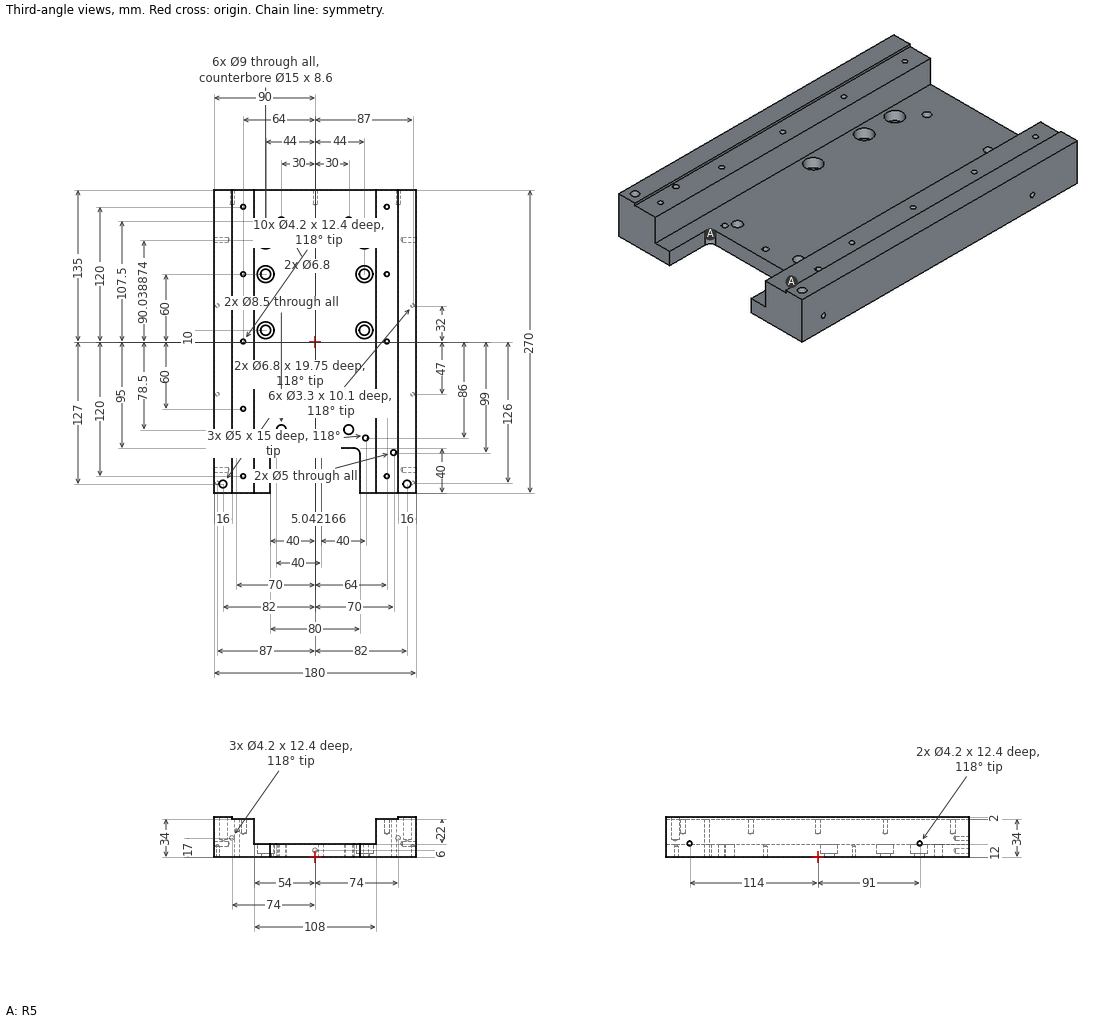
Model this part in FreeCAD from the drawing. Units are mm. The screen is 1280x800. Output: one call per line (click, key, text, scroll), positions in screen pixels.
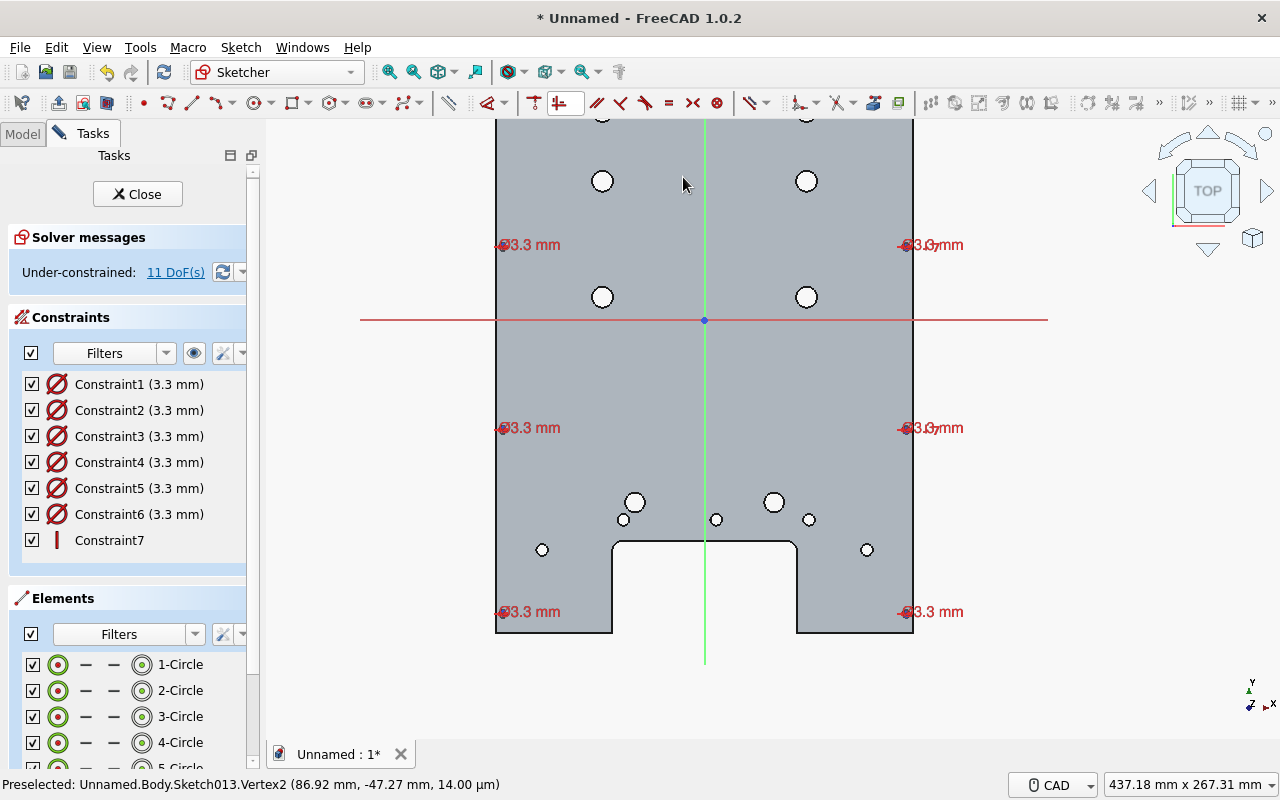
click(906, 430)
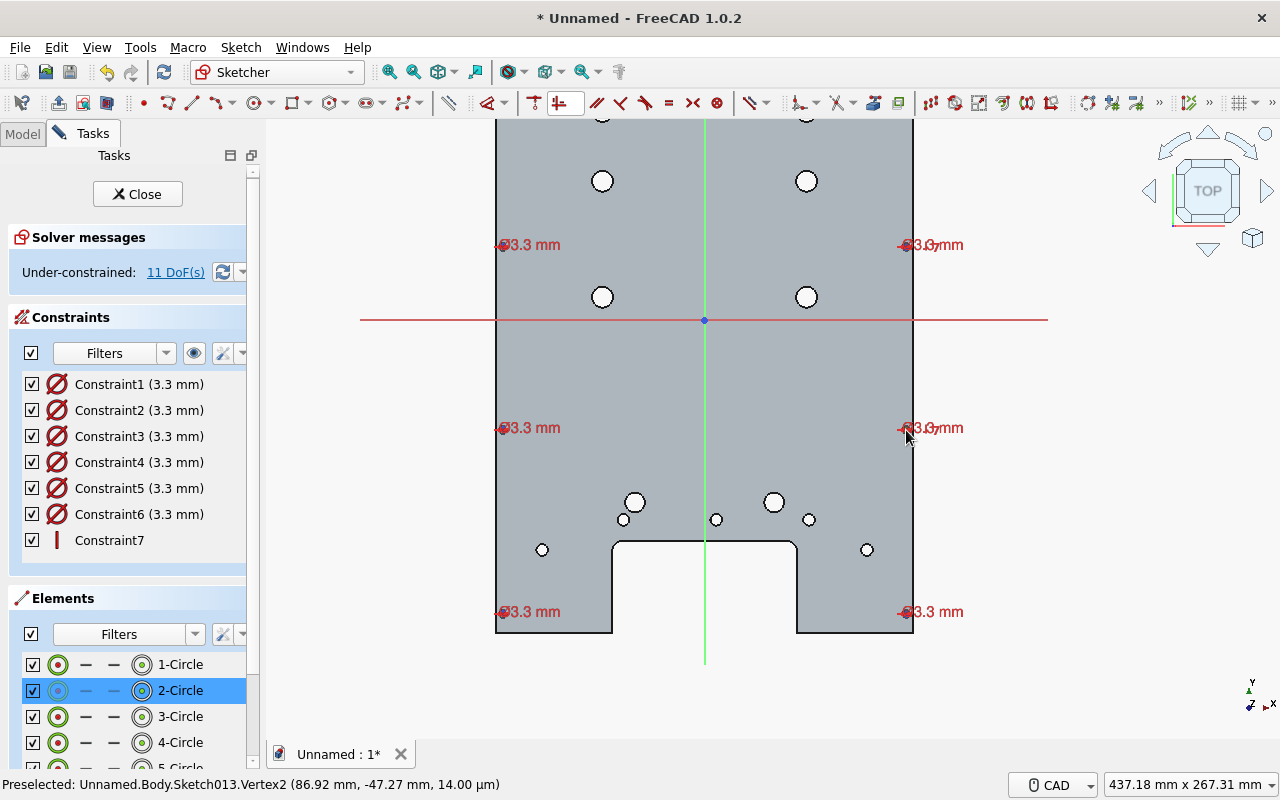
click(906, 614)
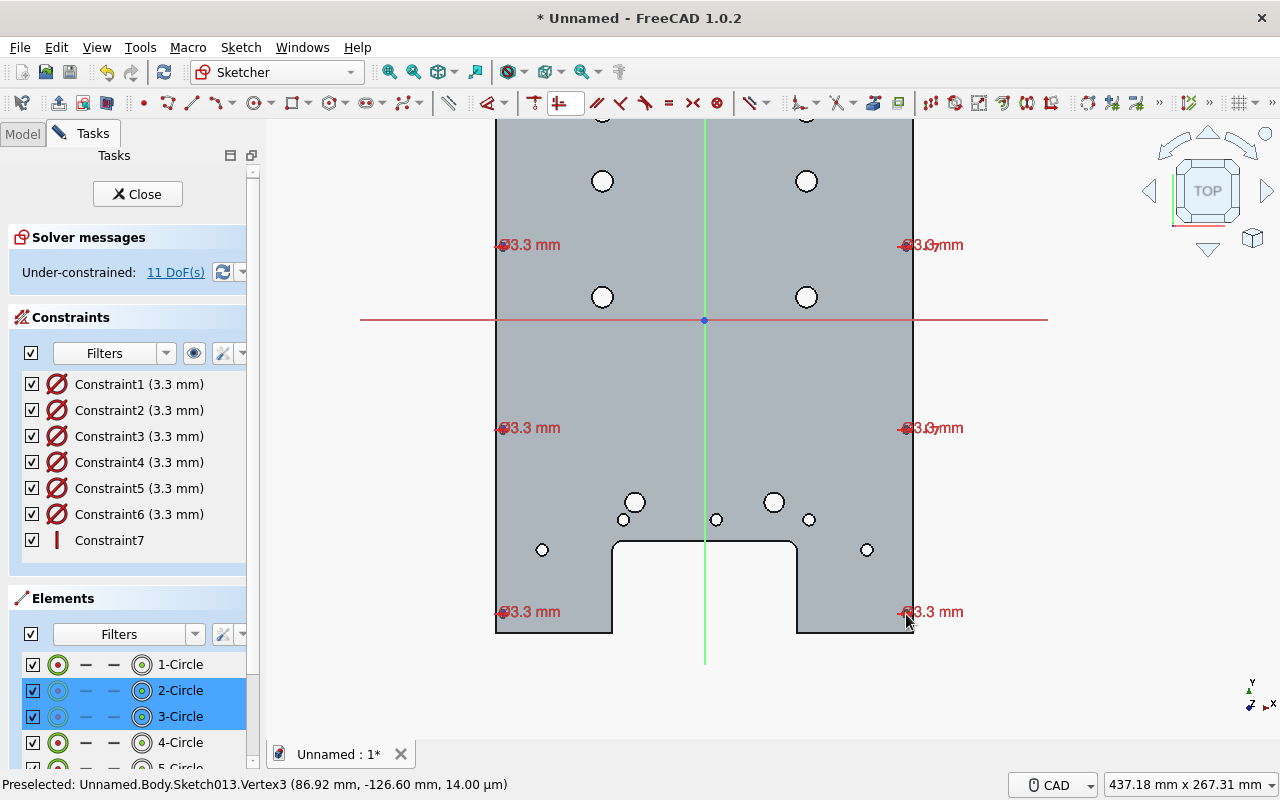
key(v)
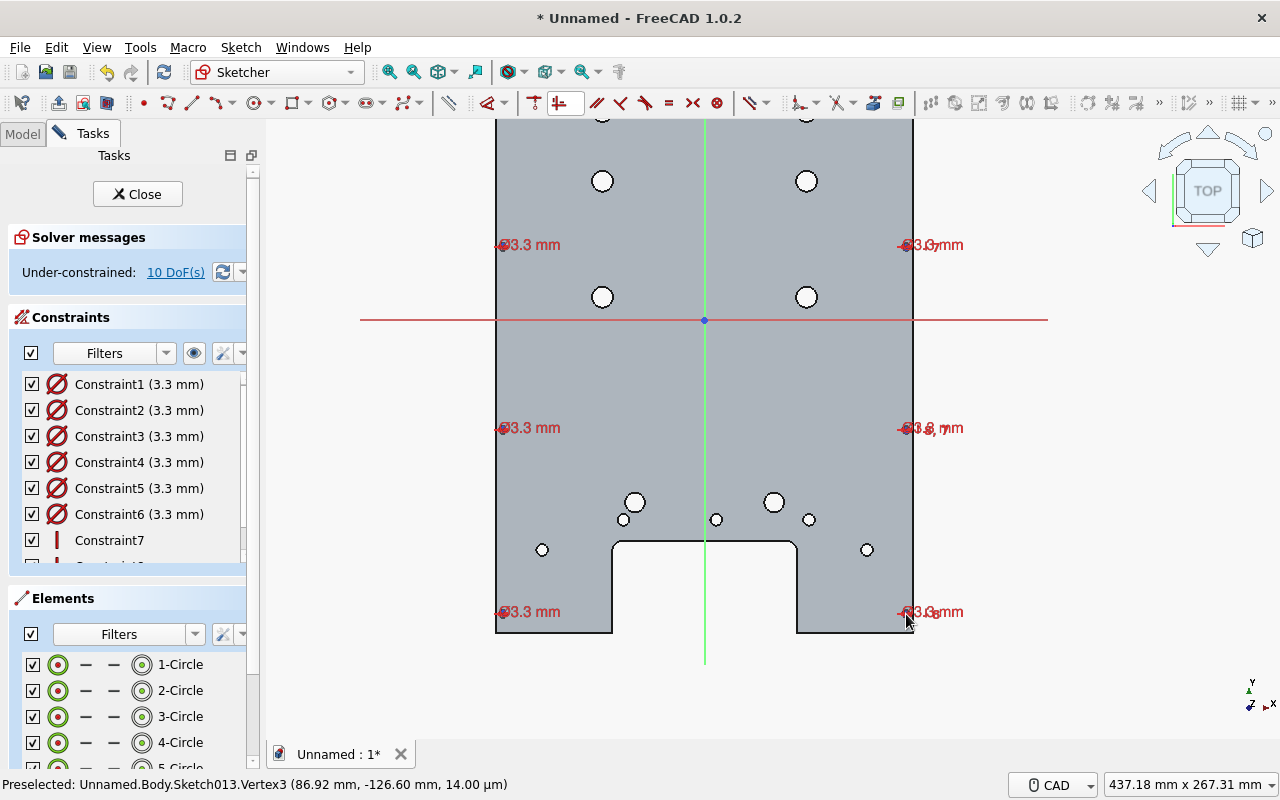
click(906, 614)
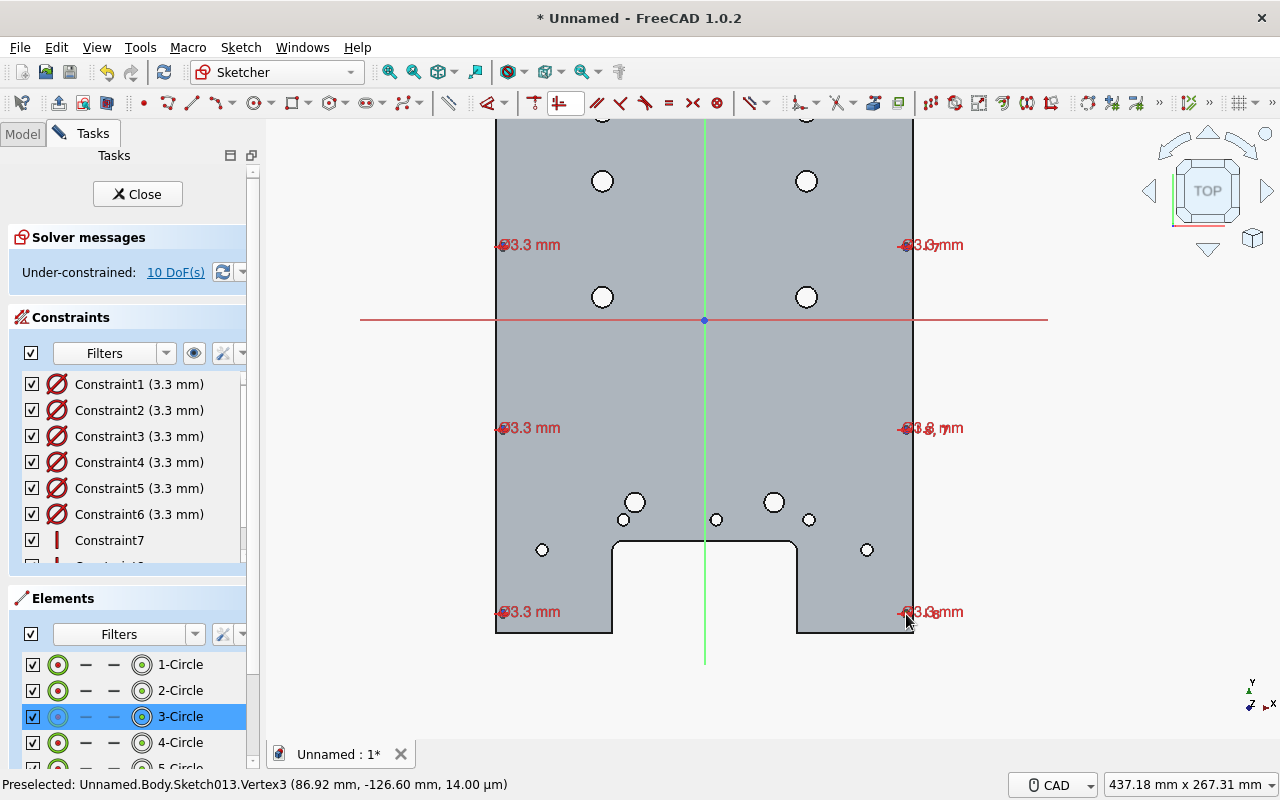
click(503, 614)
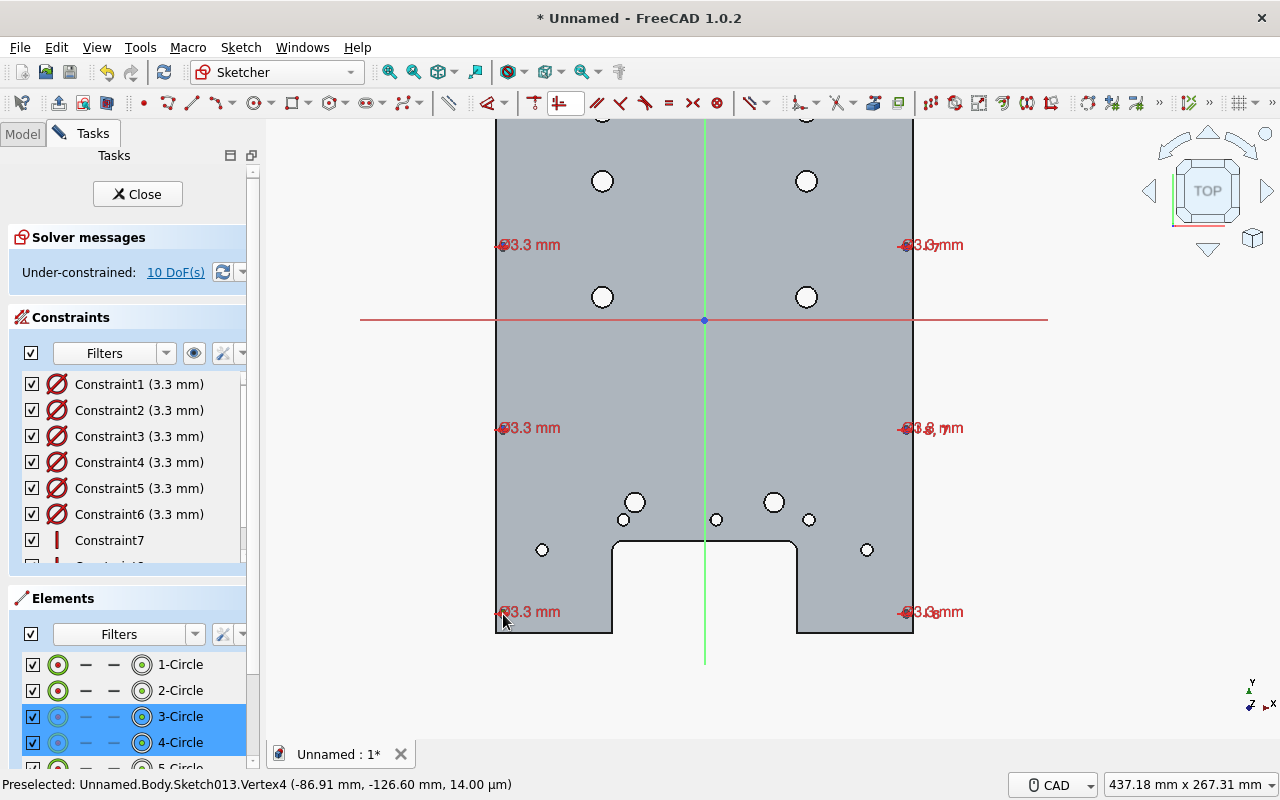
key(h)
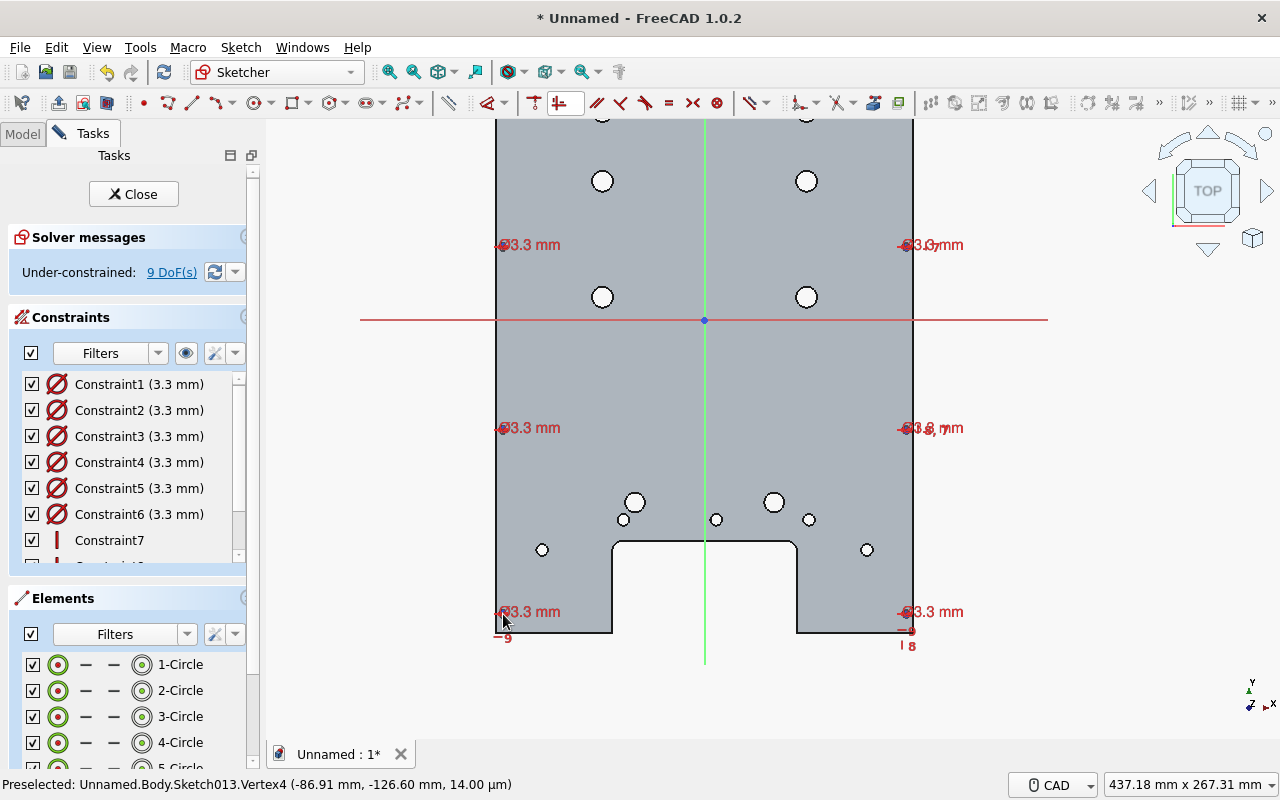
click(503, 614)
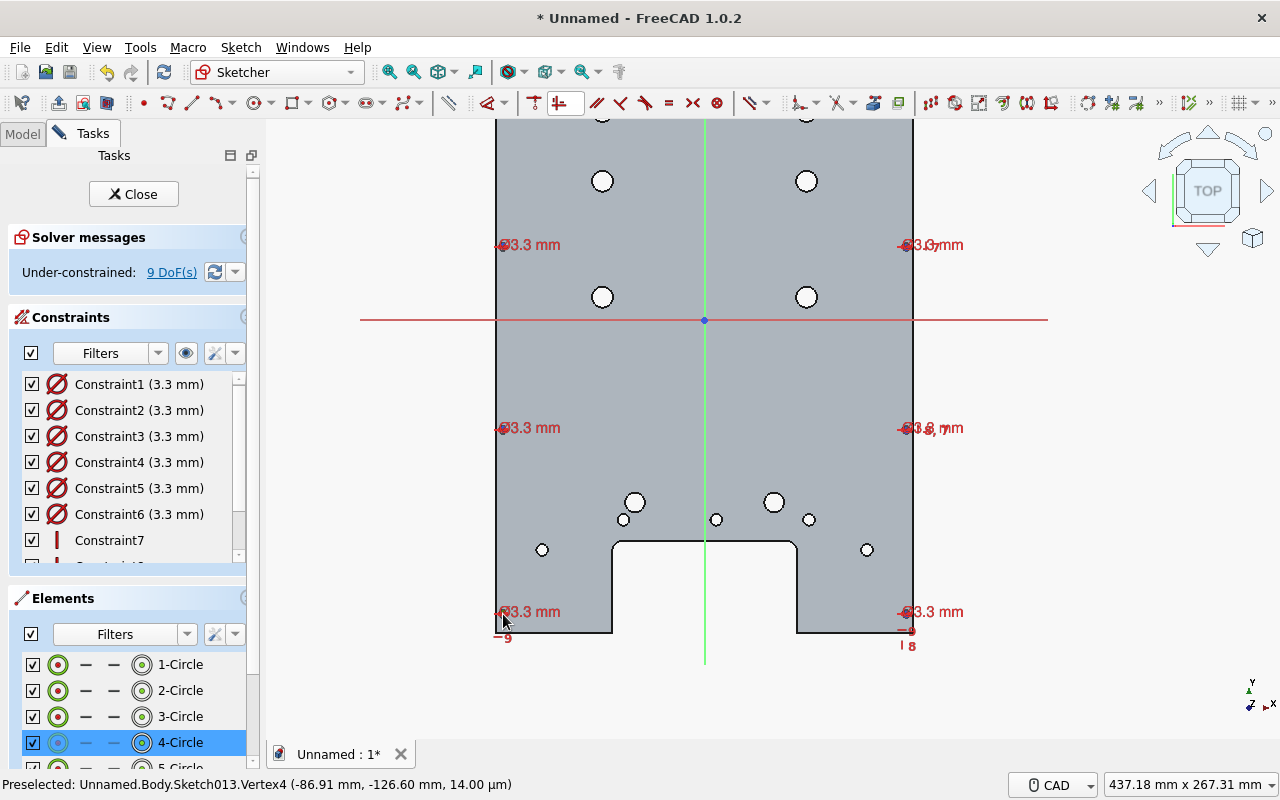
click(503, 430)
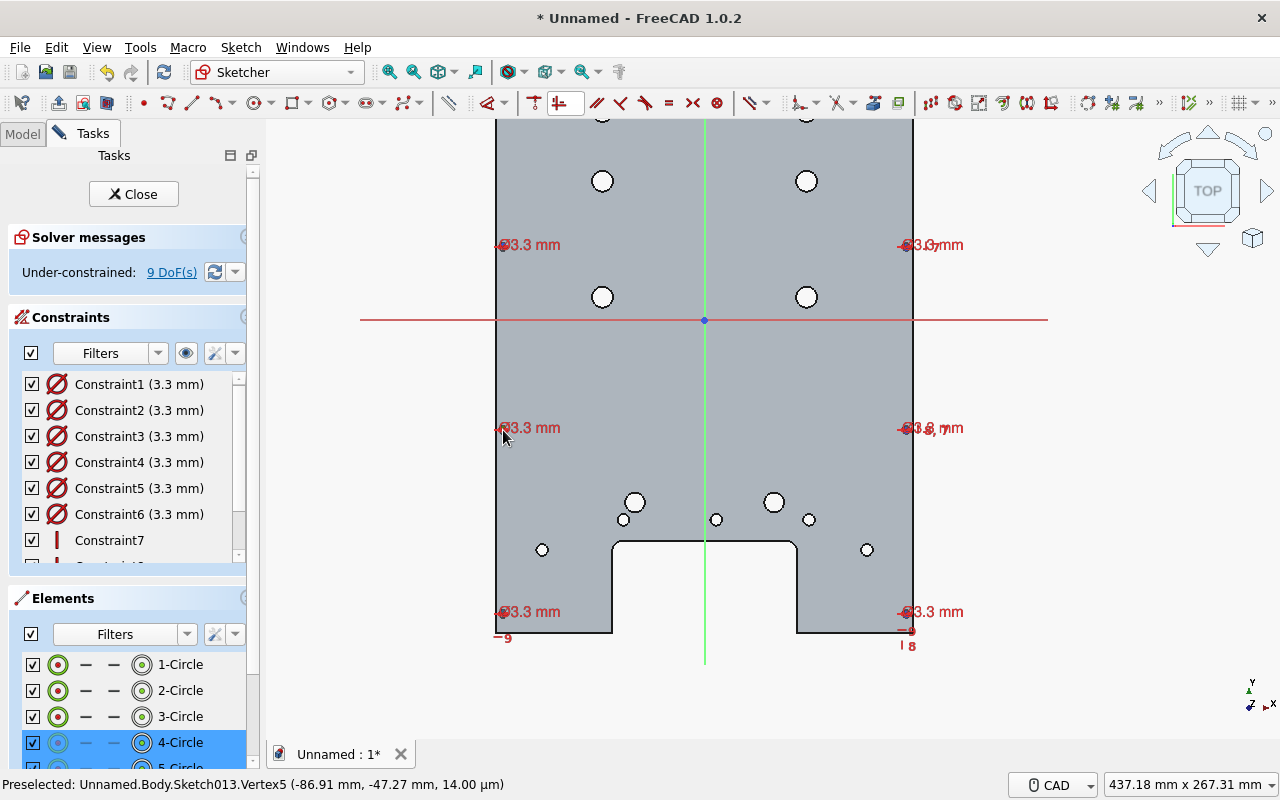
click(578, 104)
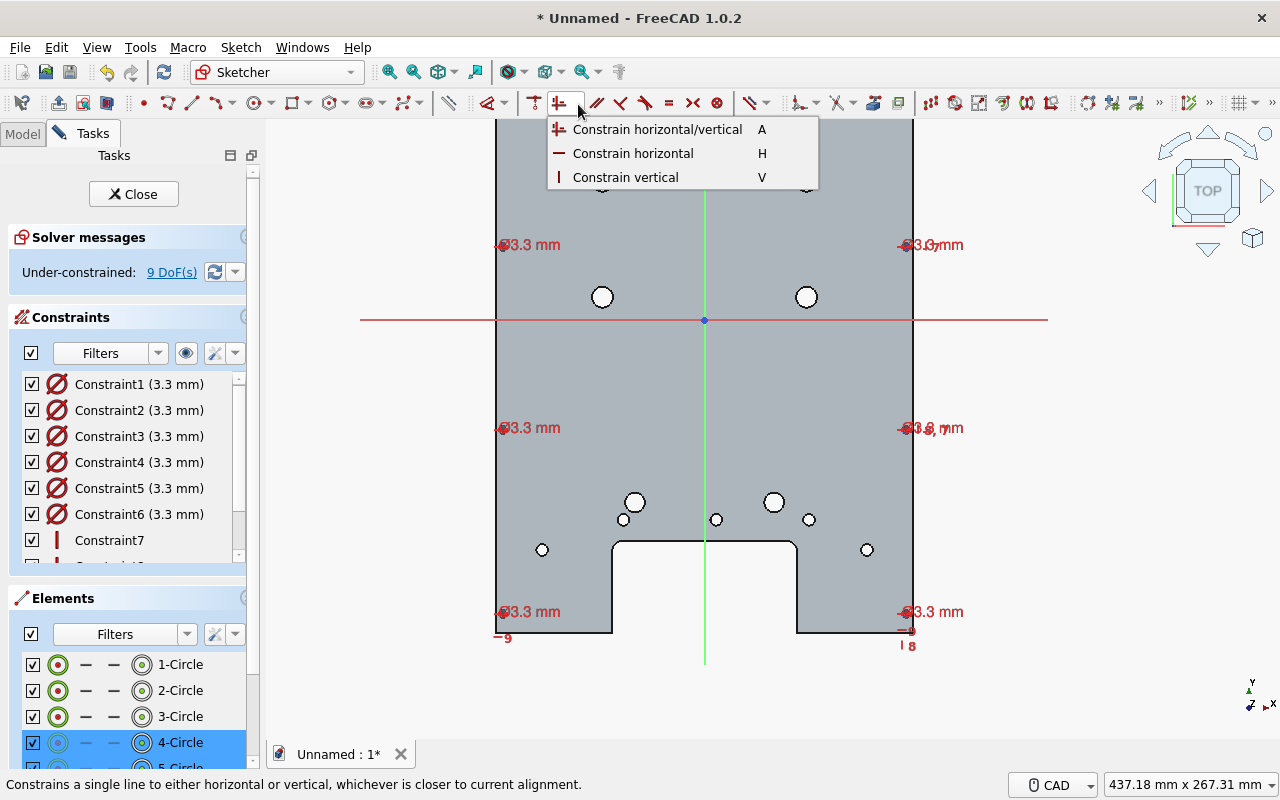
click(683, 177)